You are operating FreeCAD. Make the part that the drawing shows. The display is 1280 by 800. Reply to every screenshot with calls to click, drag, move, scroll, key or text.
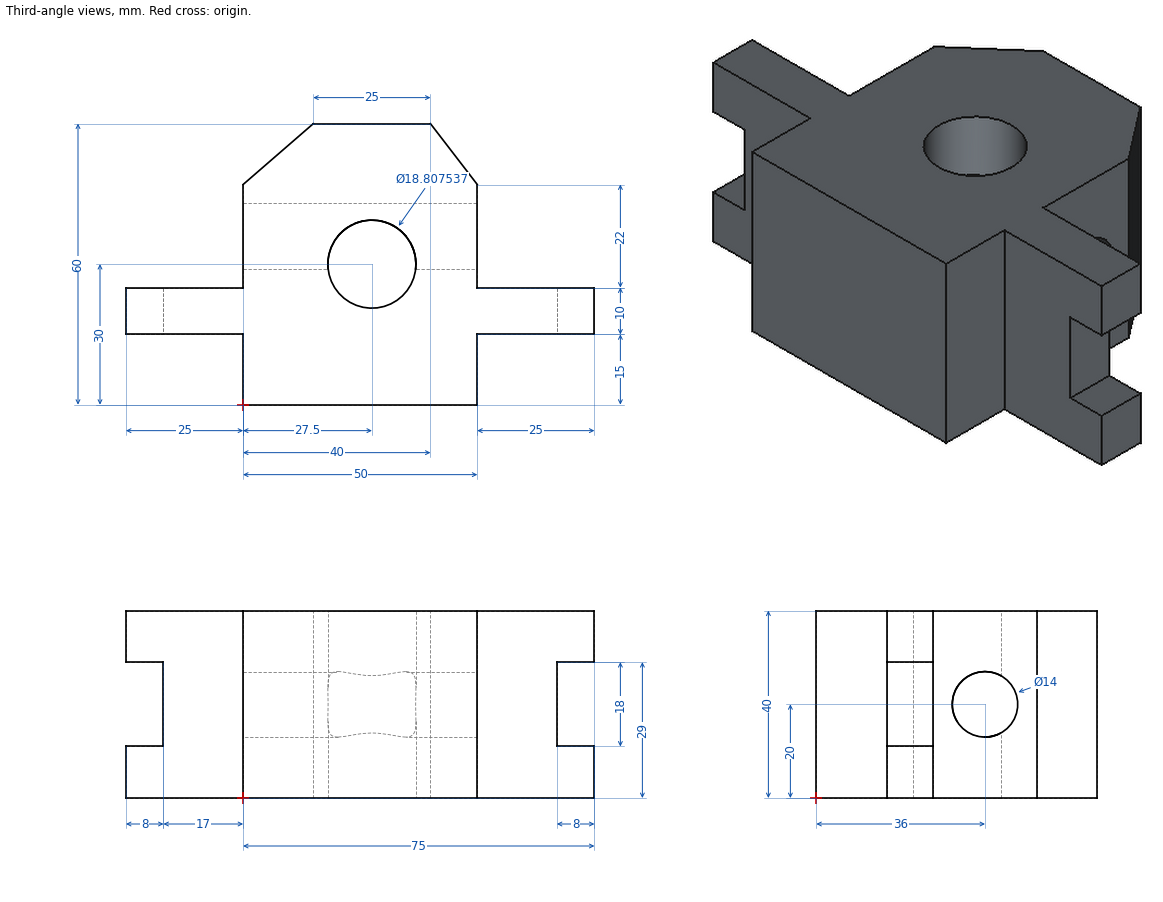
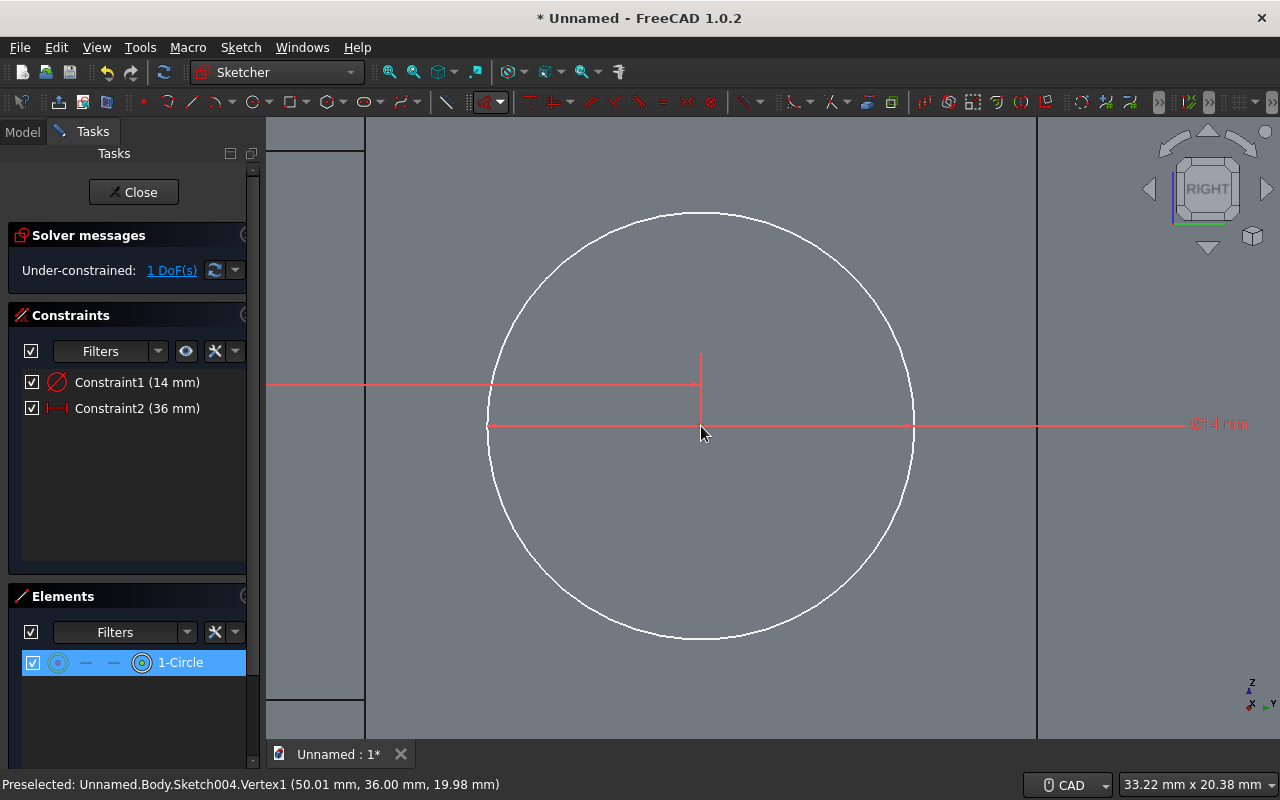
key(i)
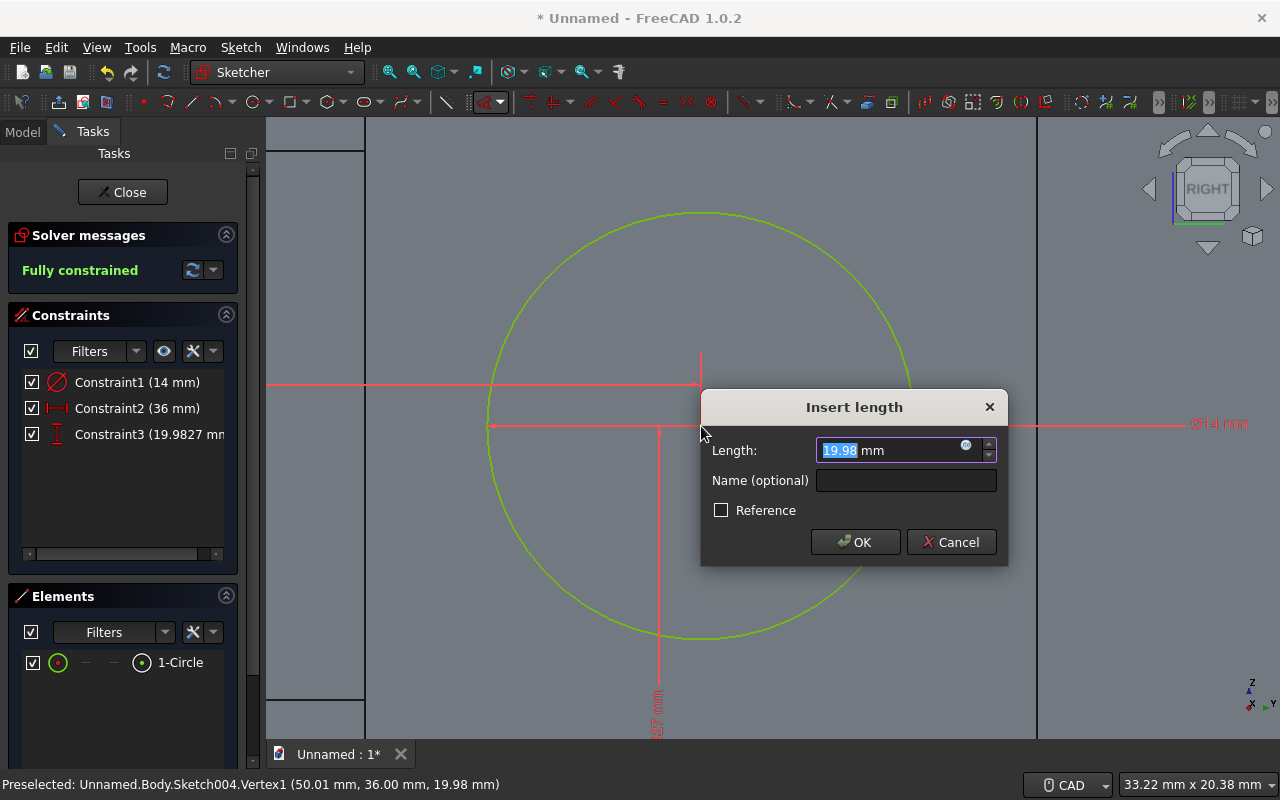
text(20)
key(Return)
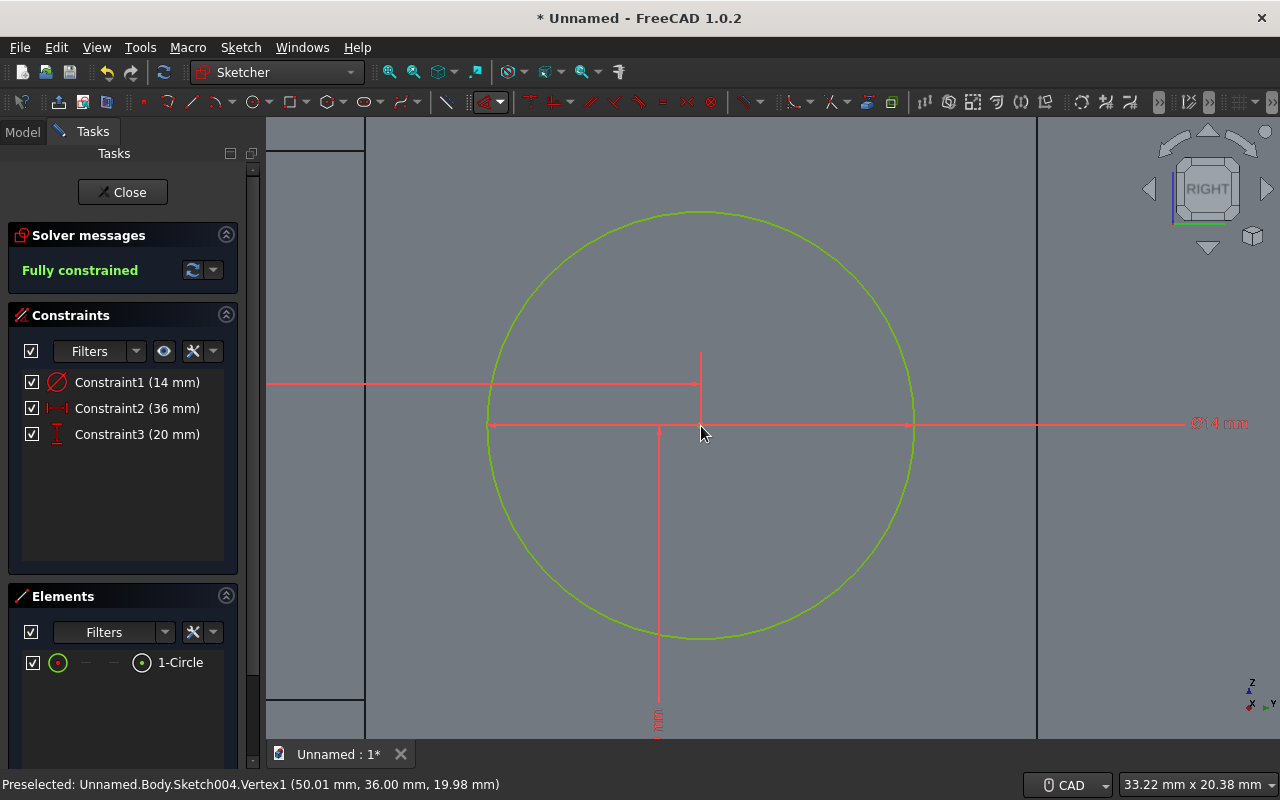
click(123, 192)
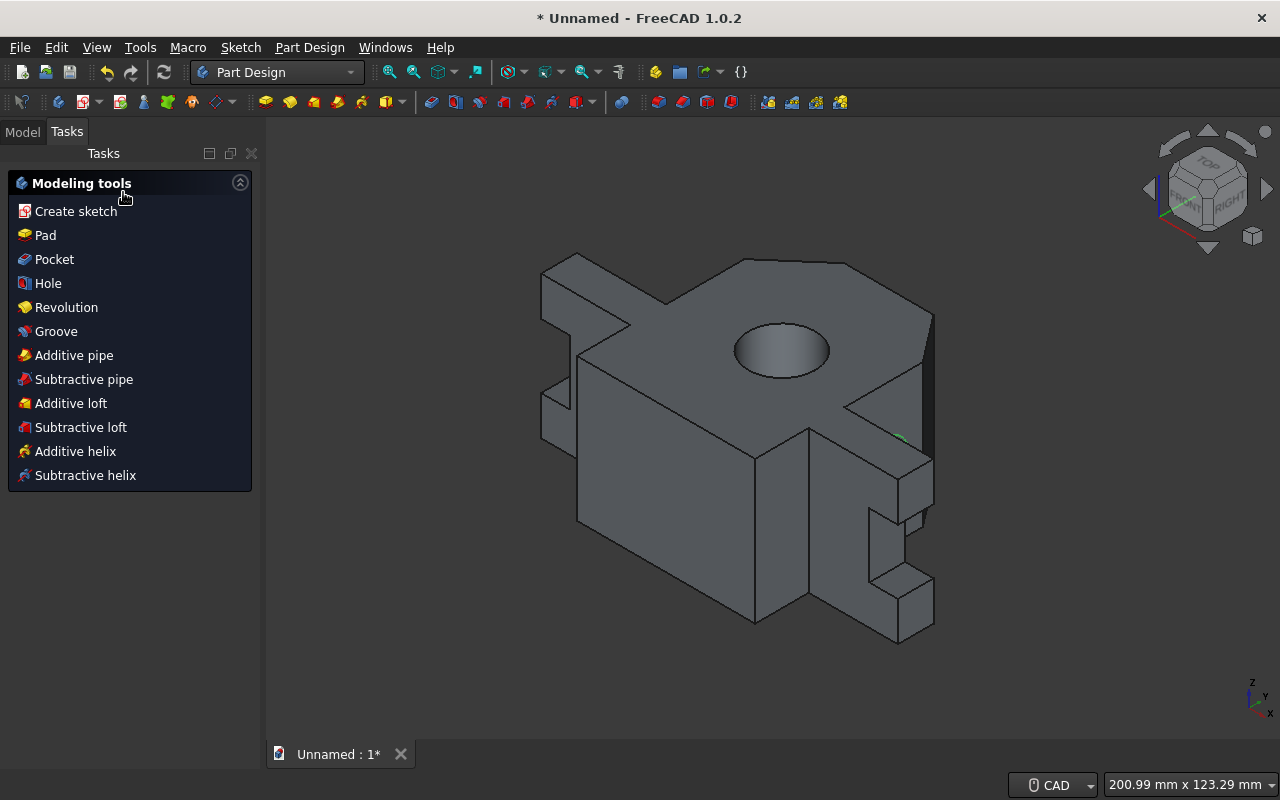
click(432, 102)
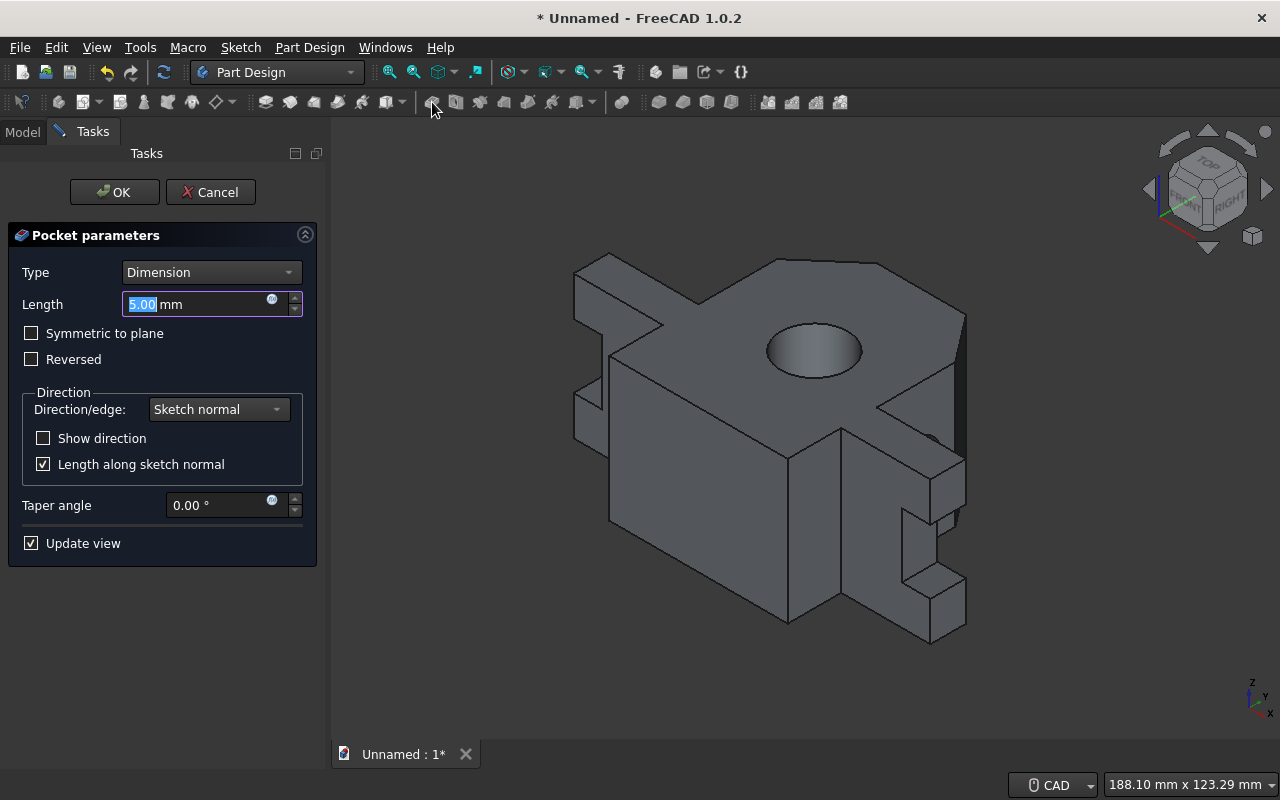
click(212, 272)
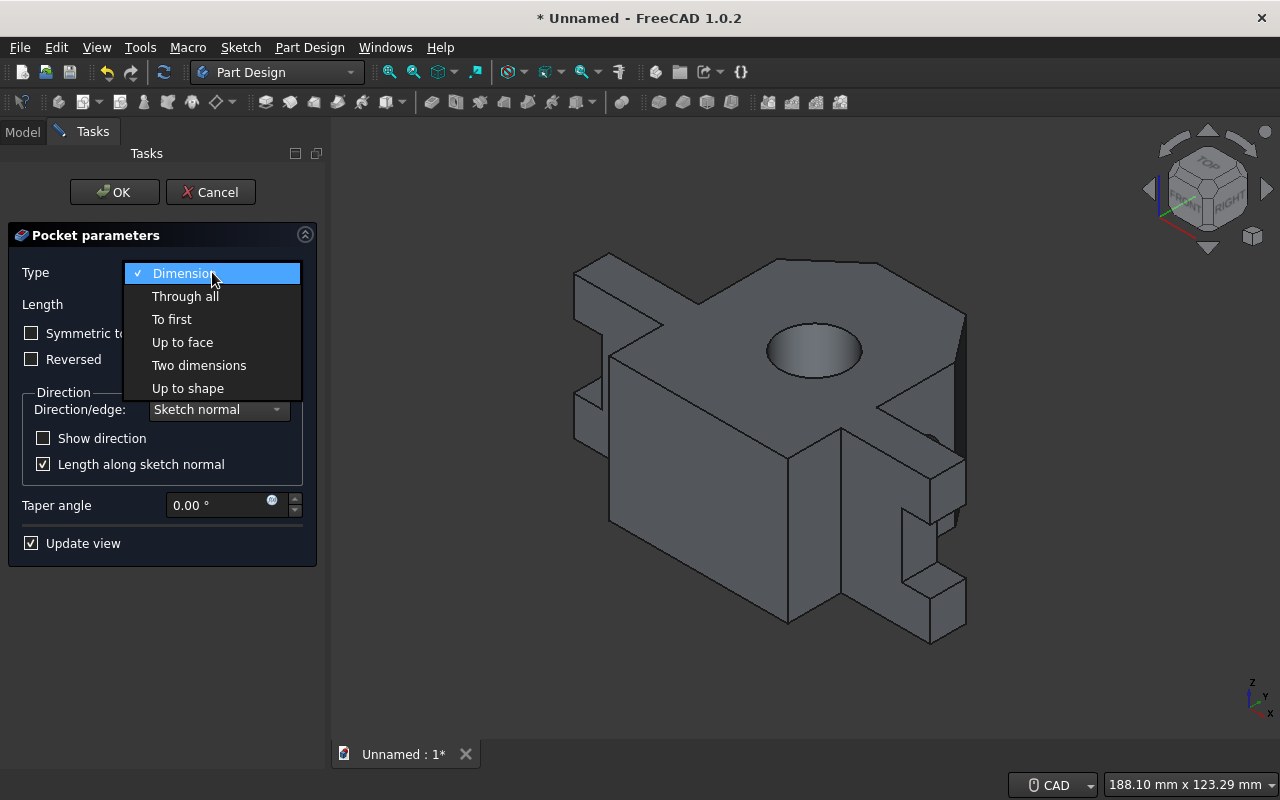
click(212, 296)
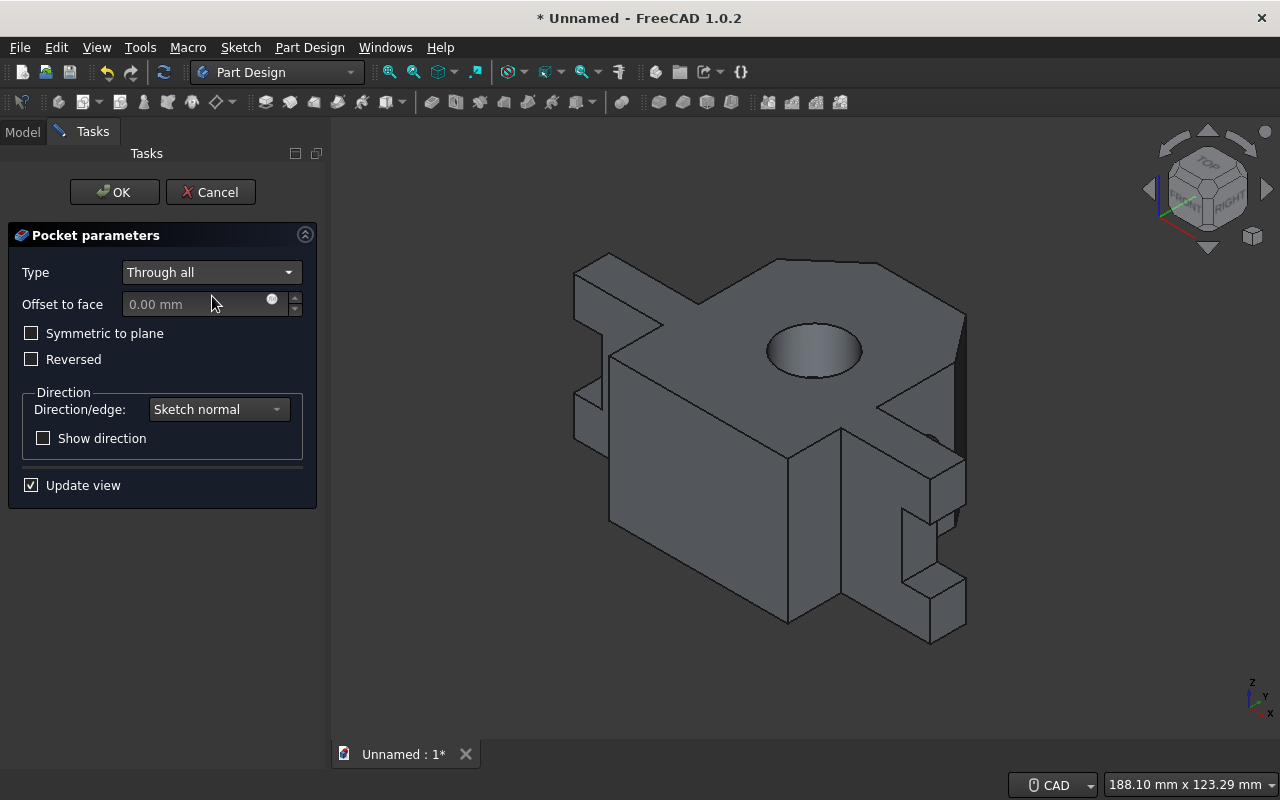
click(115, 192)